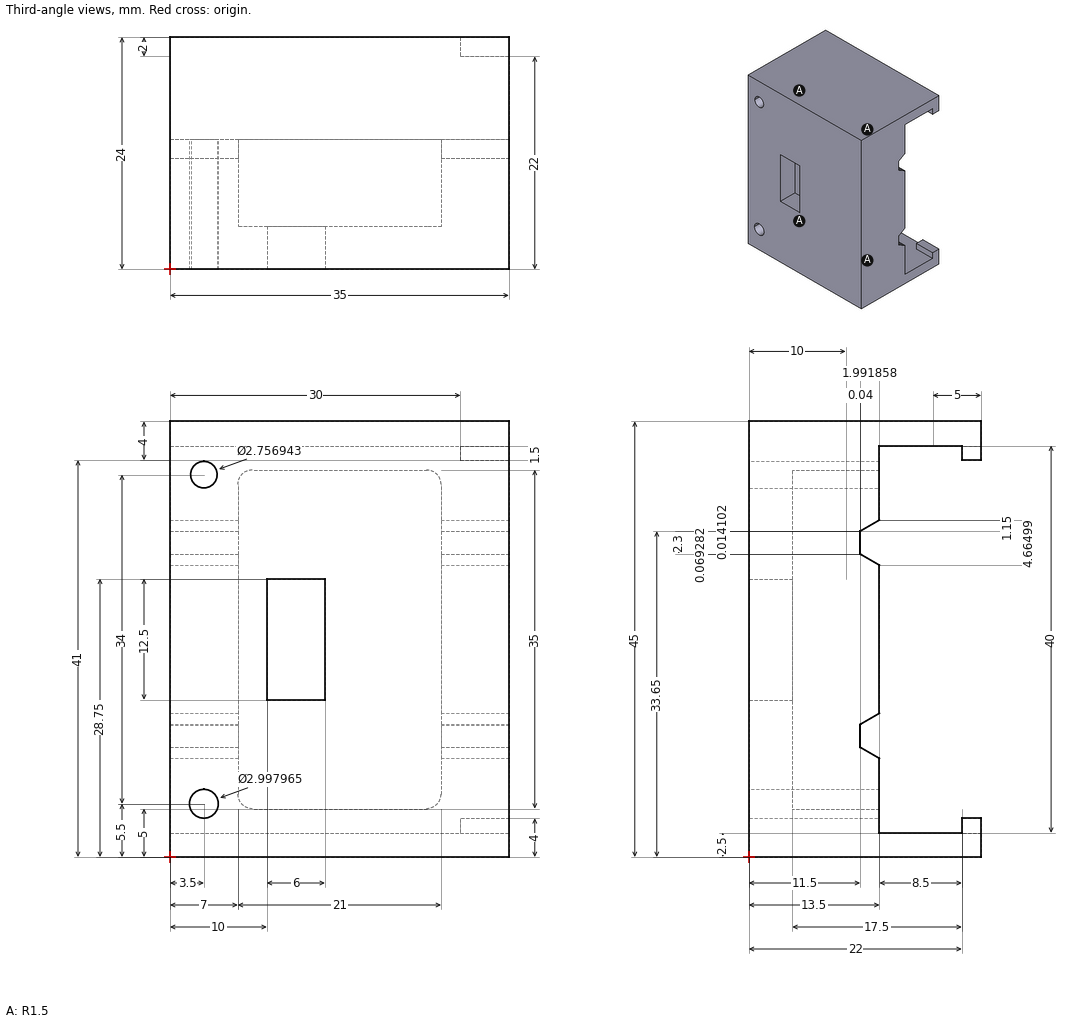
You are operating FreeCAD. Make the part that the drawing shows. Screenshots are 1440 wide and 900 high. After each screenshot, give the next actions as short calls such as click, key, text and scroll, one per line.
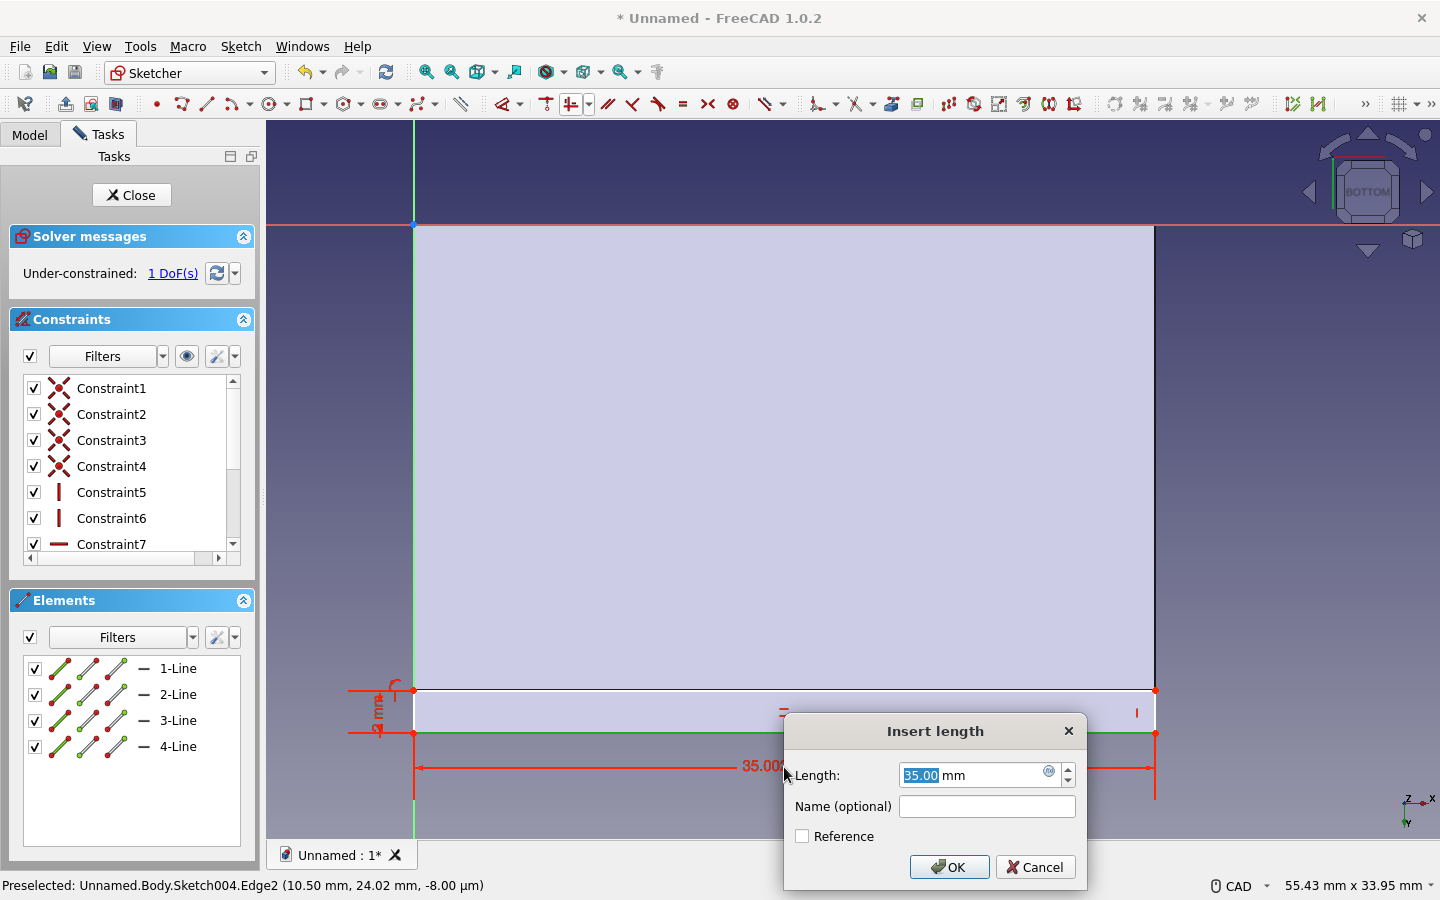
text(35)
key(Return)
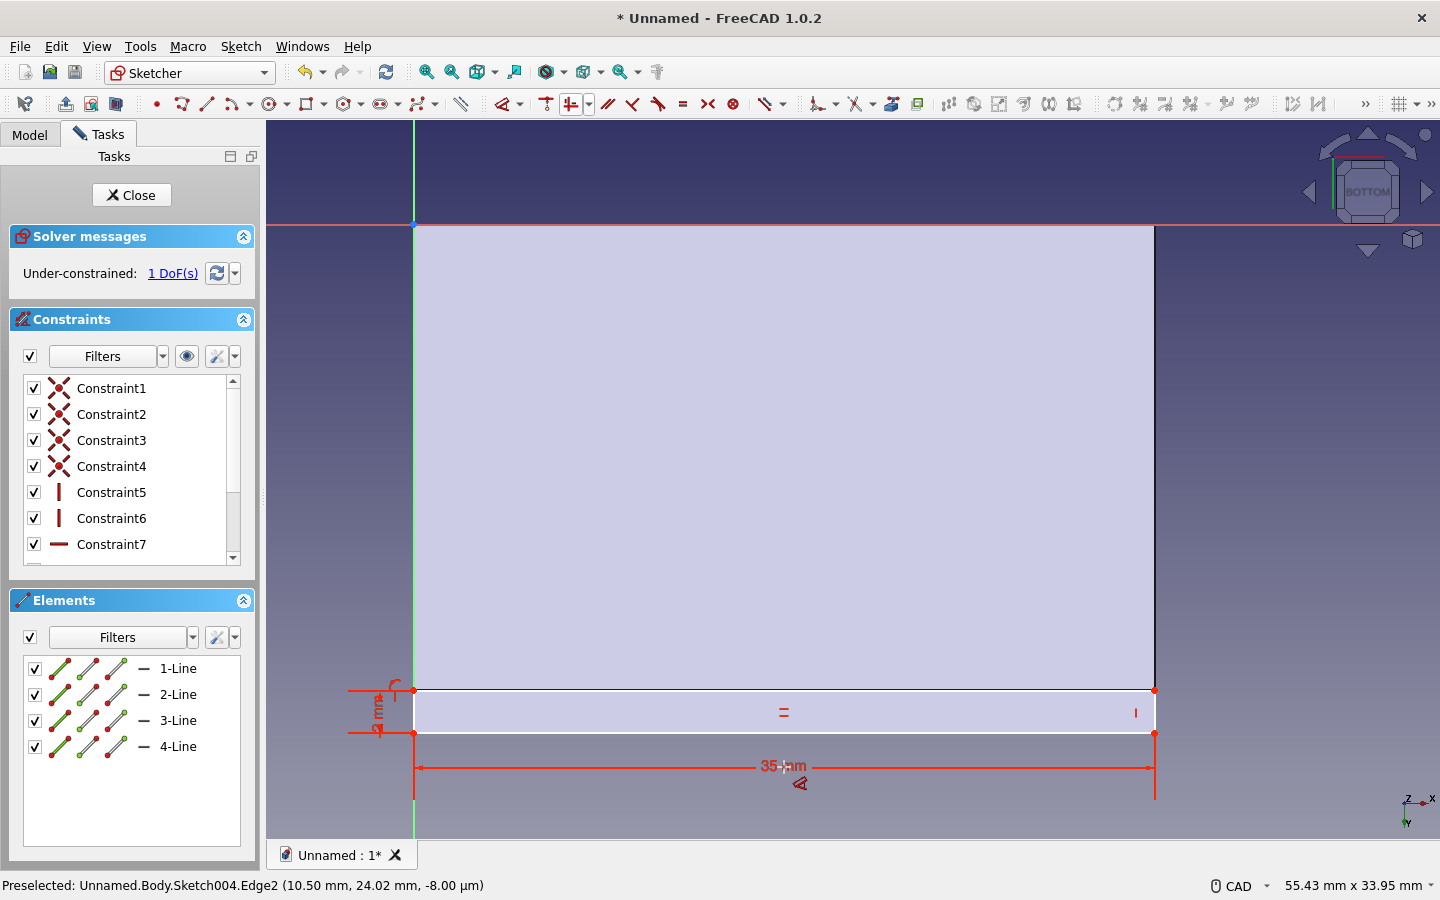
click(414, 691)
click(380, 458)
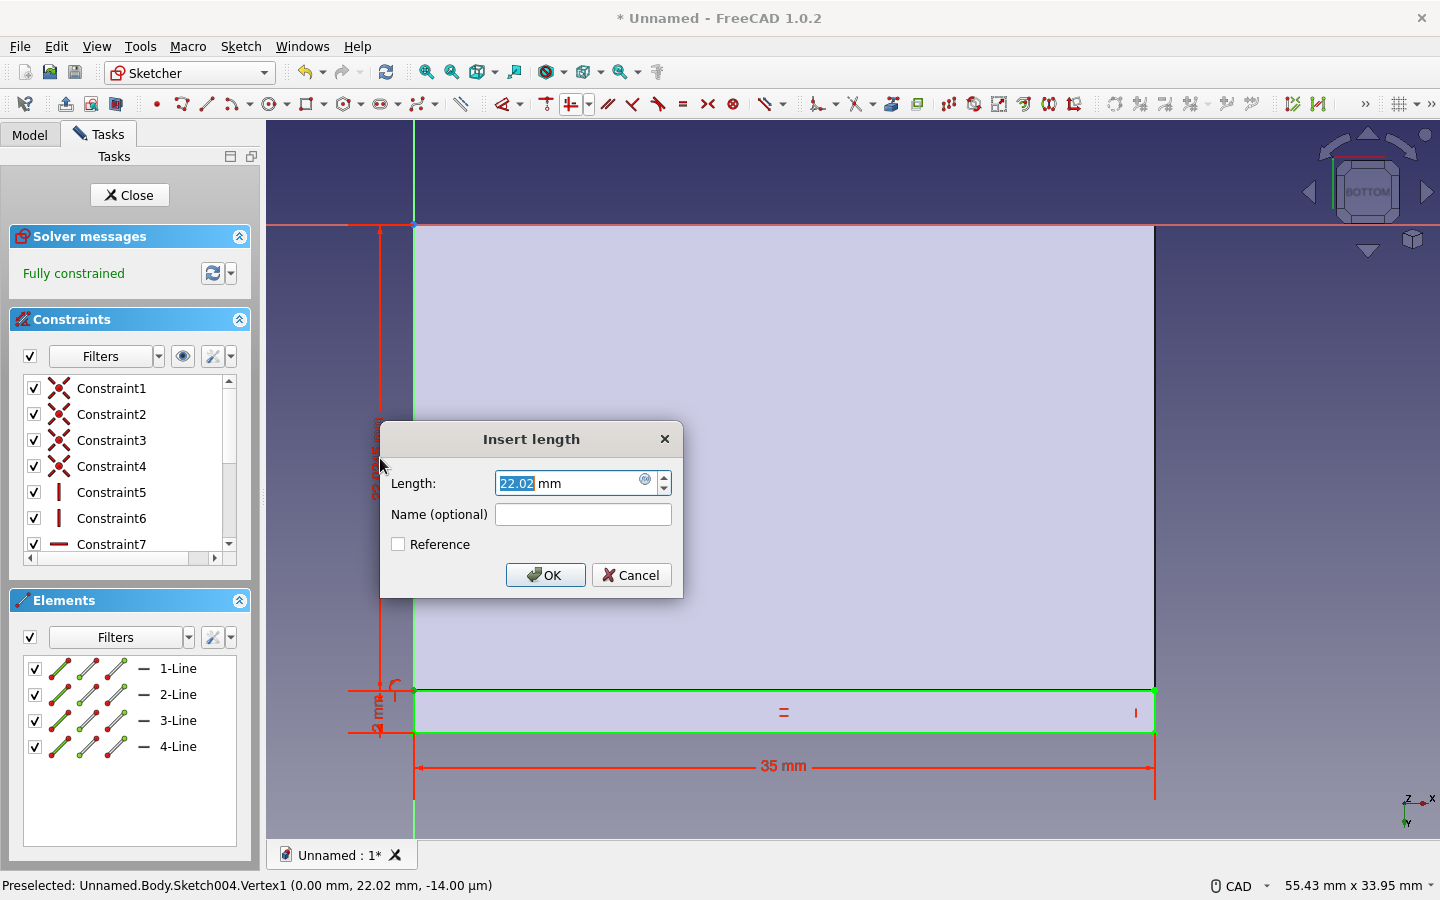
text(22)
key(Return)
key(Escape)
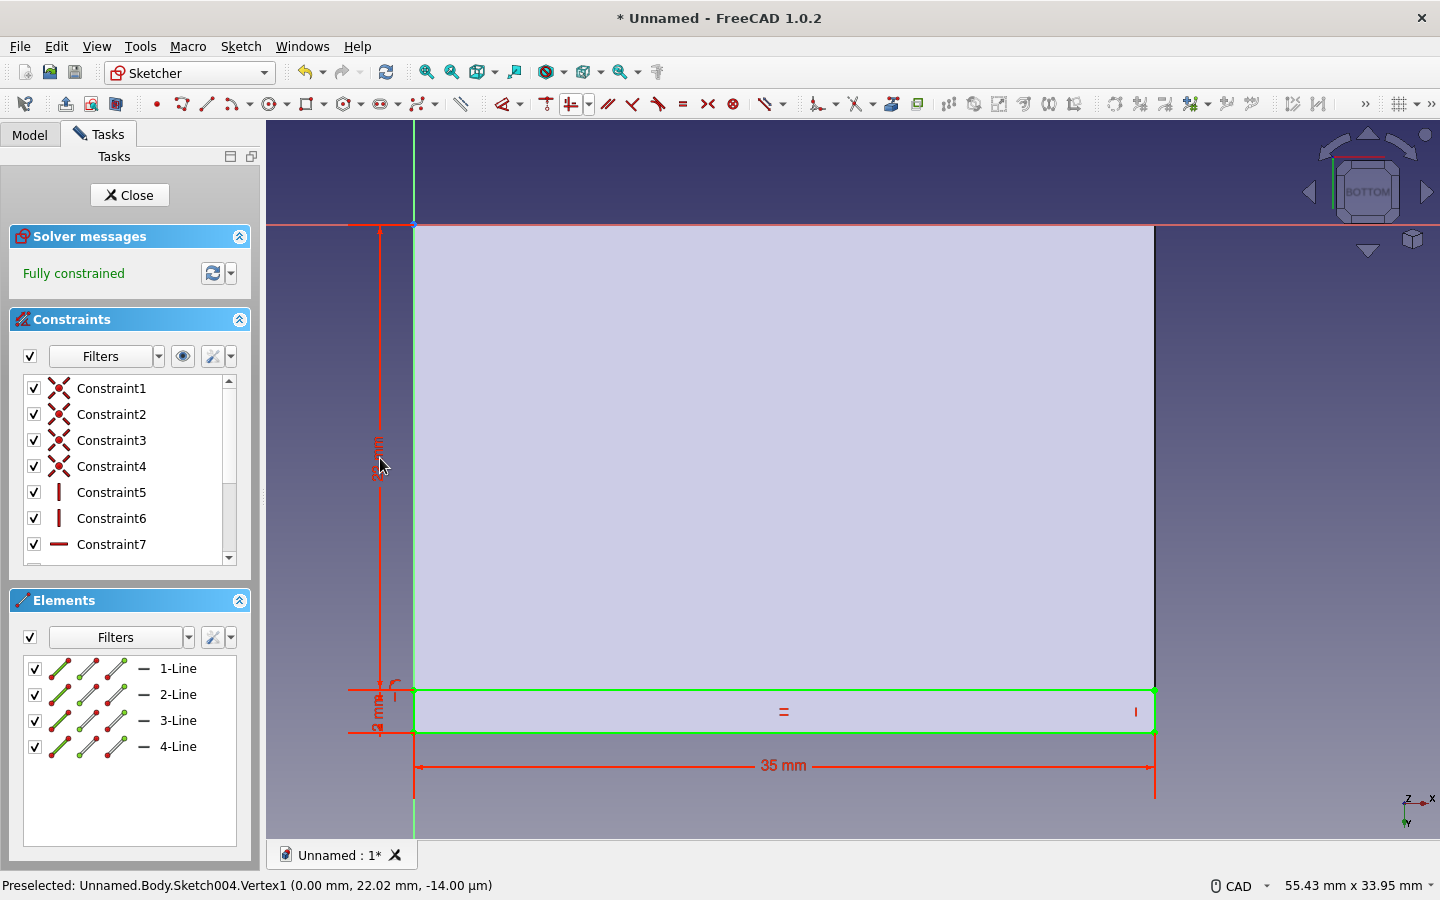
click(130, 195)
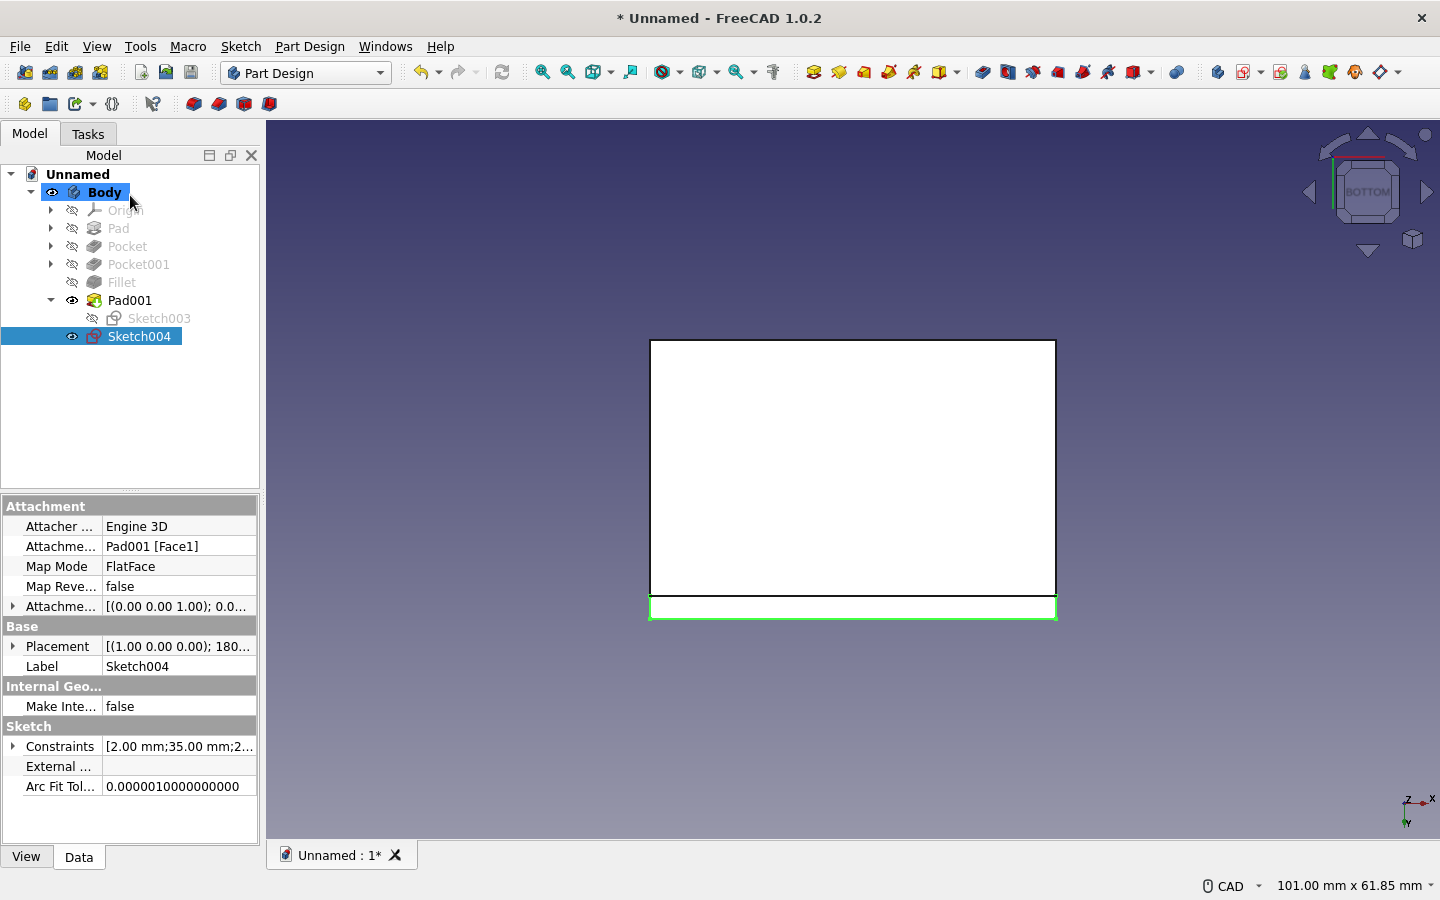
click(814, 72)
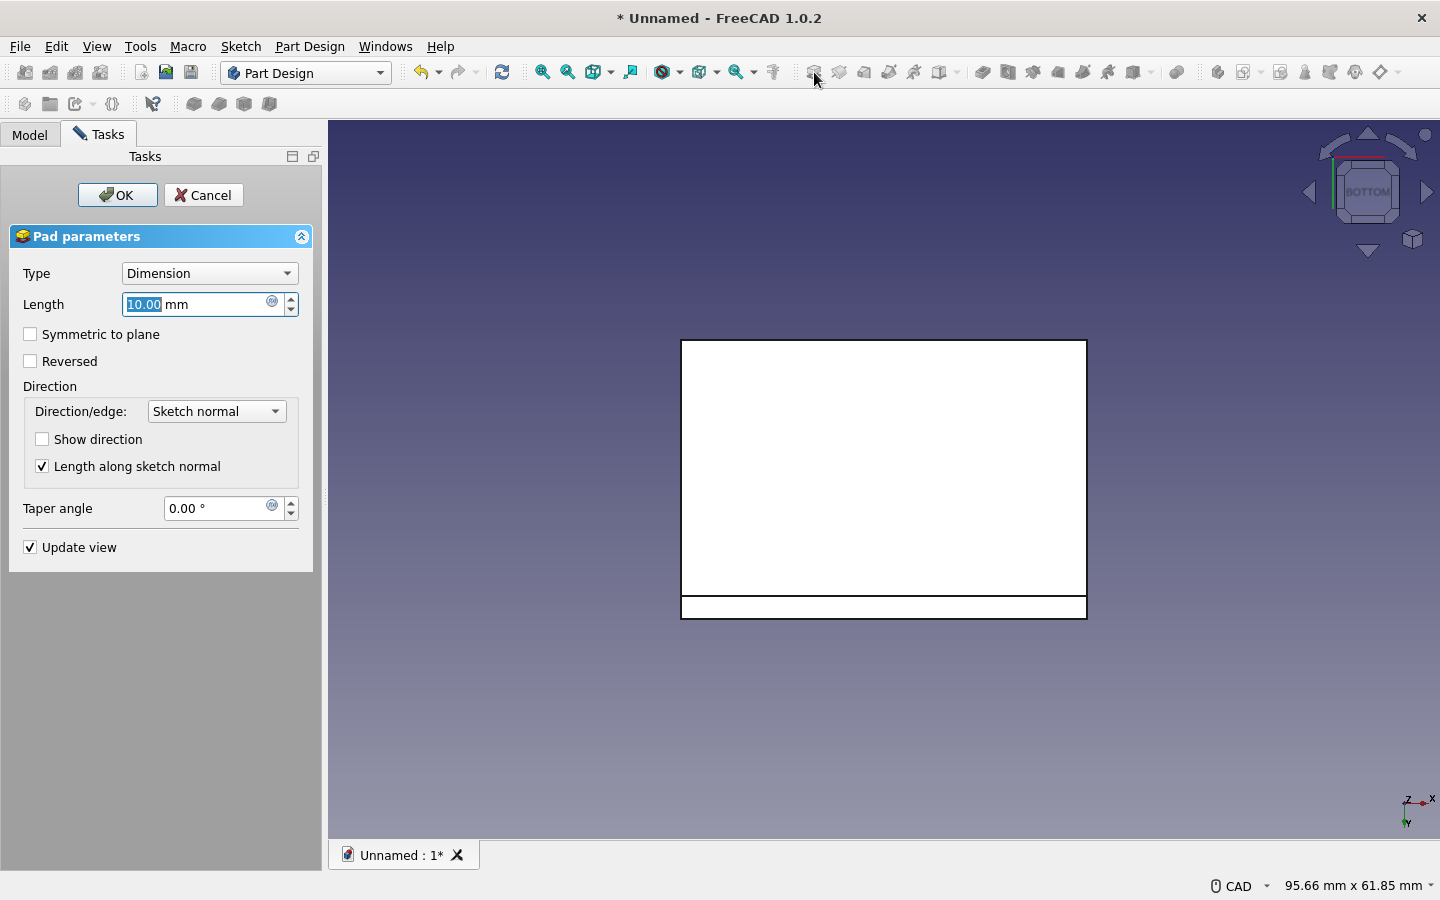
text(4)
key(Tab)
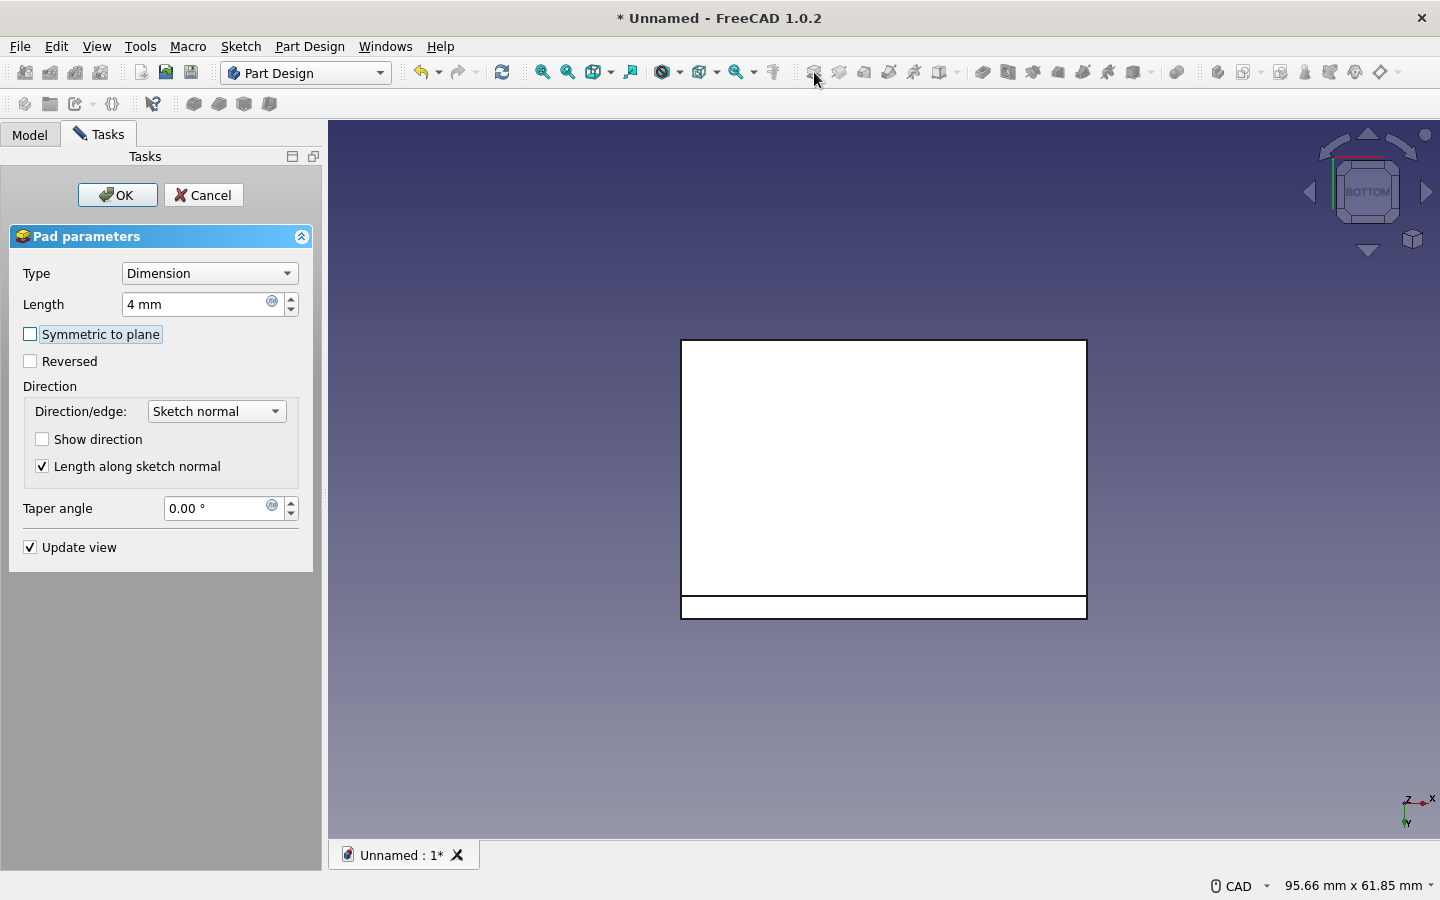
click(31, 361)